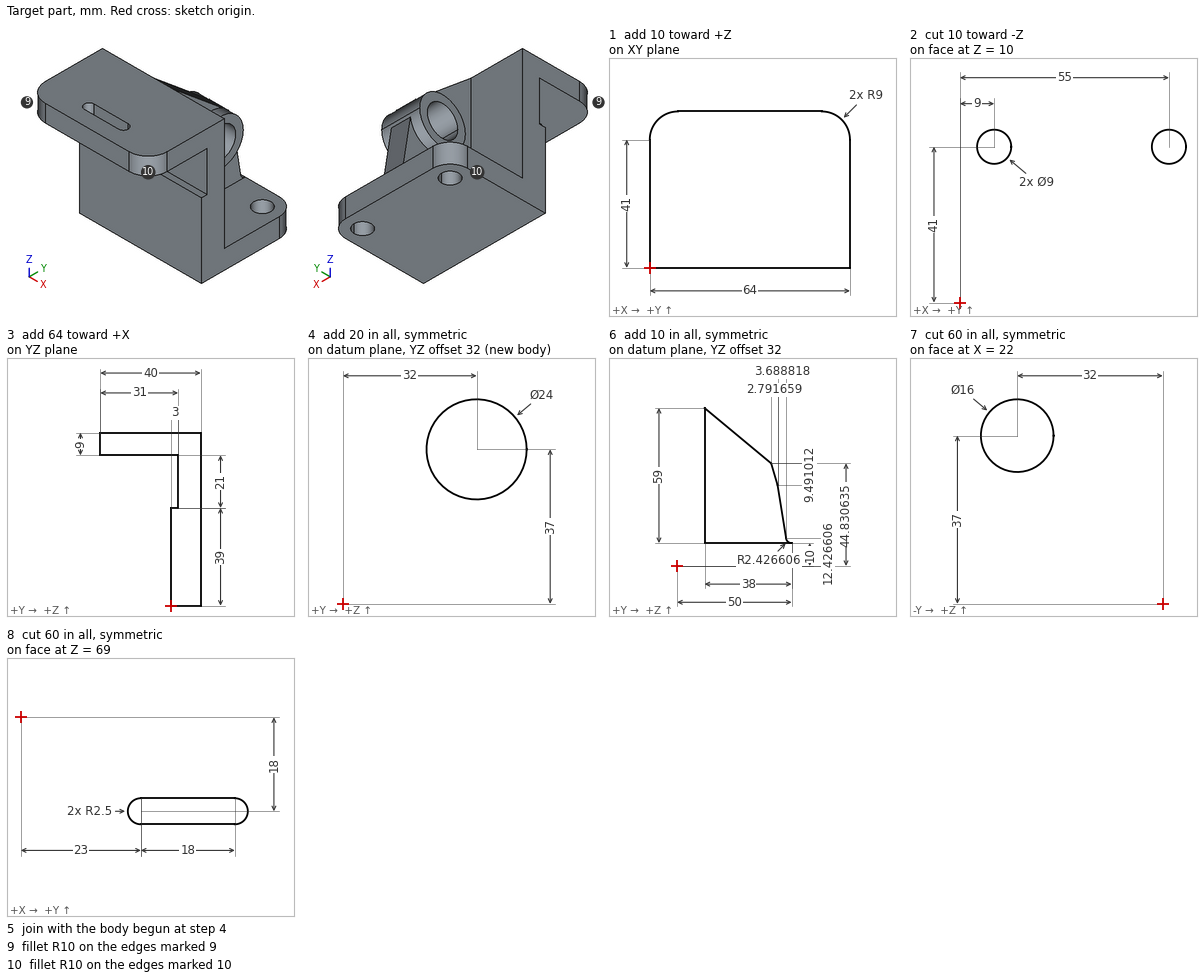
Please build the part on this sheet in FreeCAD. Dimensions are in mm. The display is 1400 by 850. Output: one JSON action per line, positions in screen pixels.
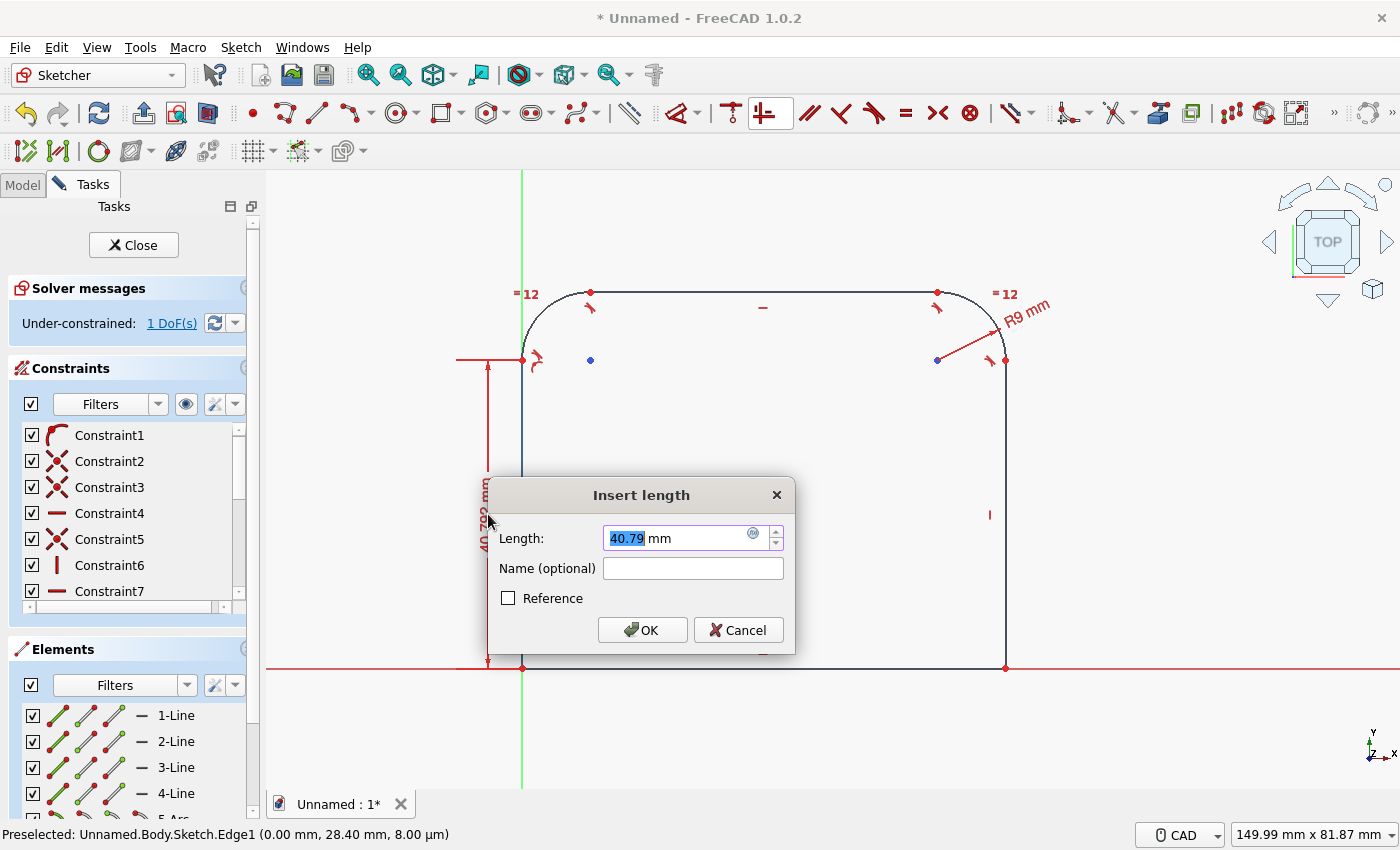
{"action": "type", "text": "41"}
{"action": "key", "text": "Return"}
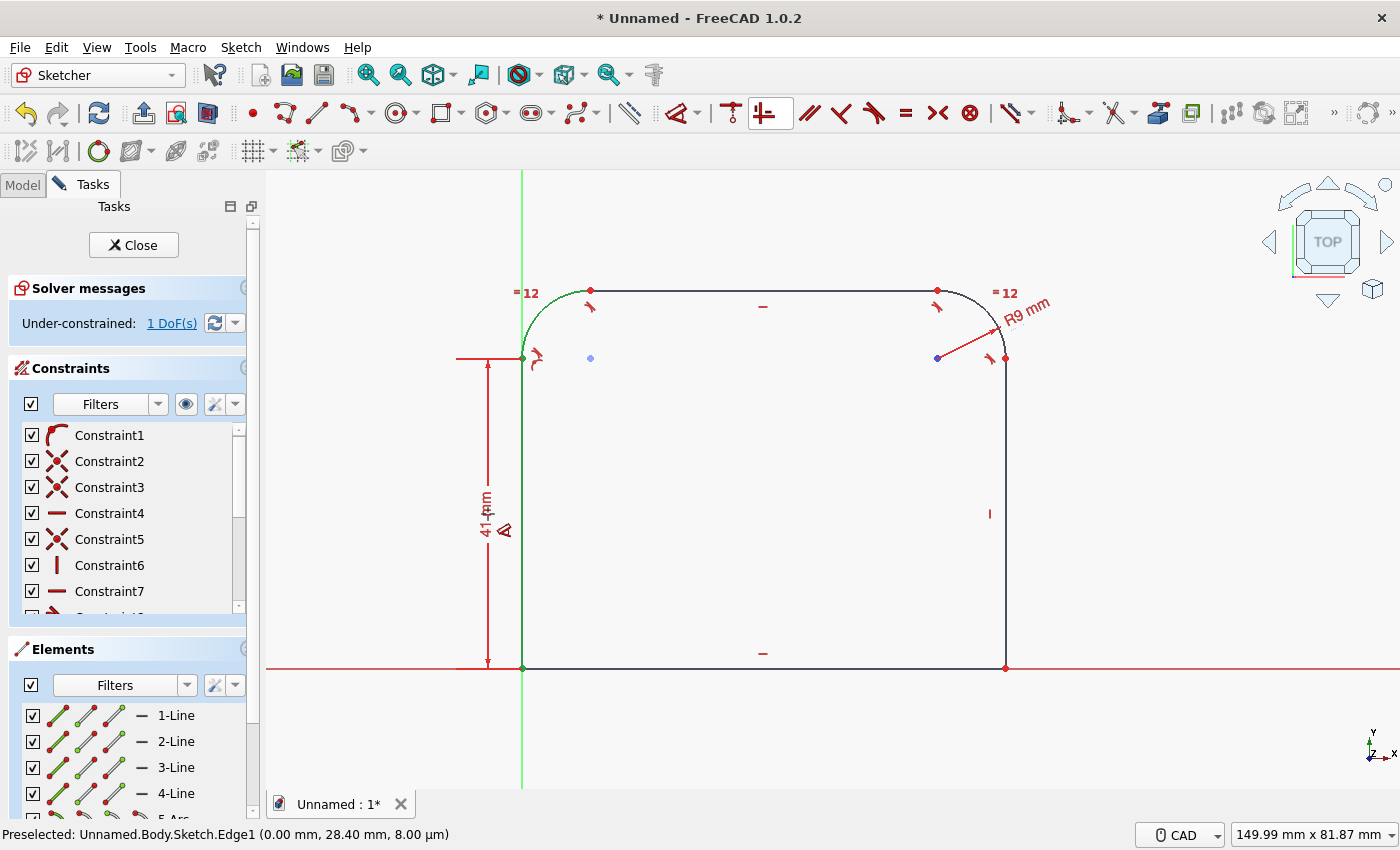
{"action": "left_click", "coordinate": [667, 669]}
{"action": "left_click", "coordinate": [764, 703]}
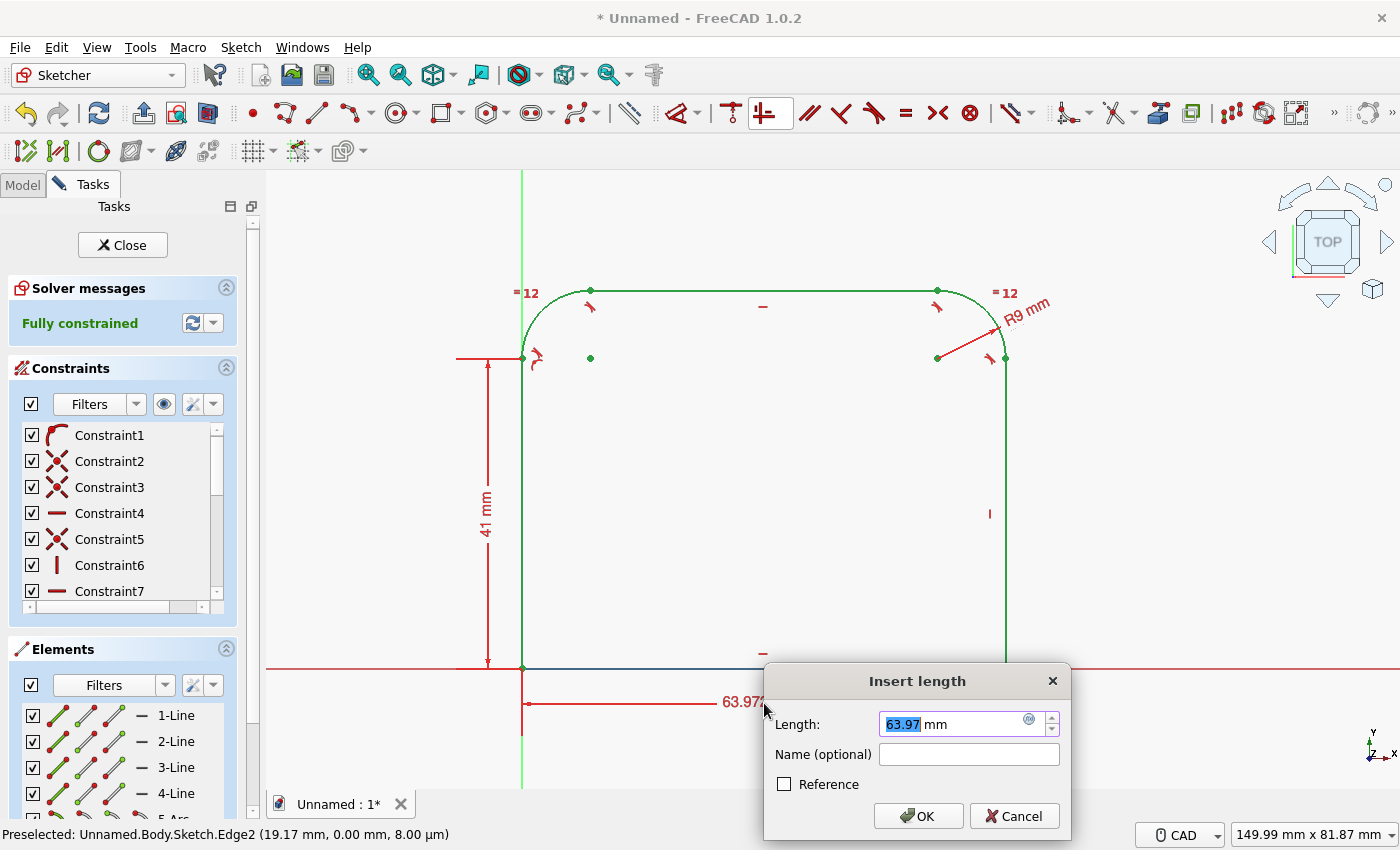
{"action": "type", "text": "64"}
{"action": "key", "text": "Return"}
{"action": "key", "text": "Escape"}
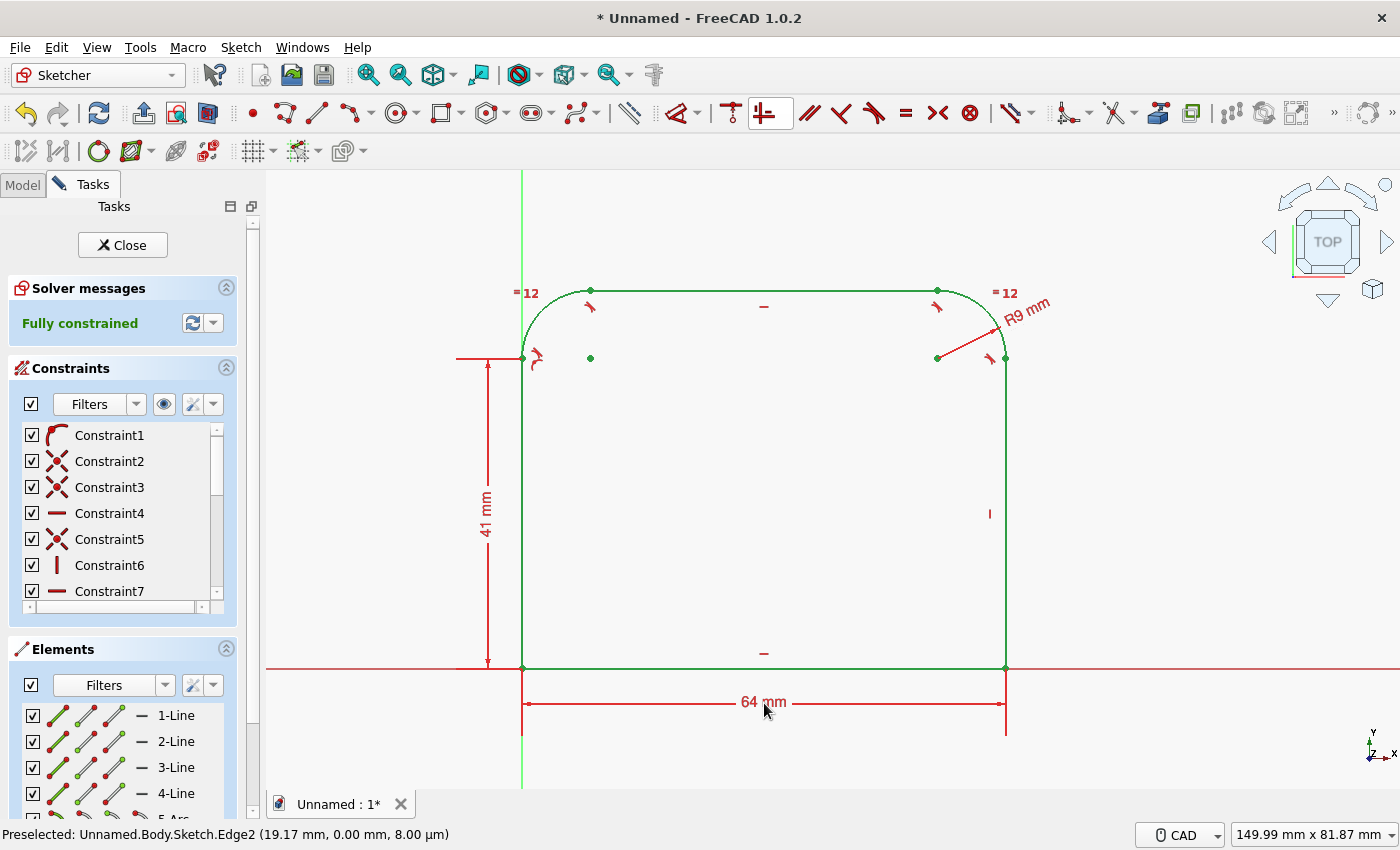
{"action": "left_click", "coordinate": [123, 245]}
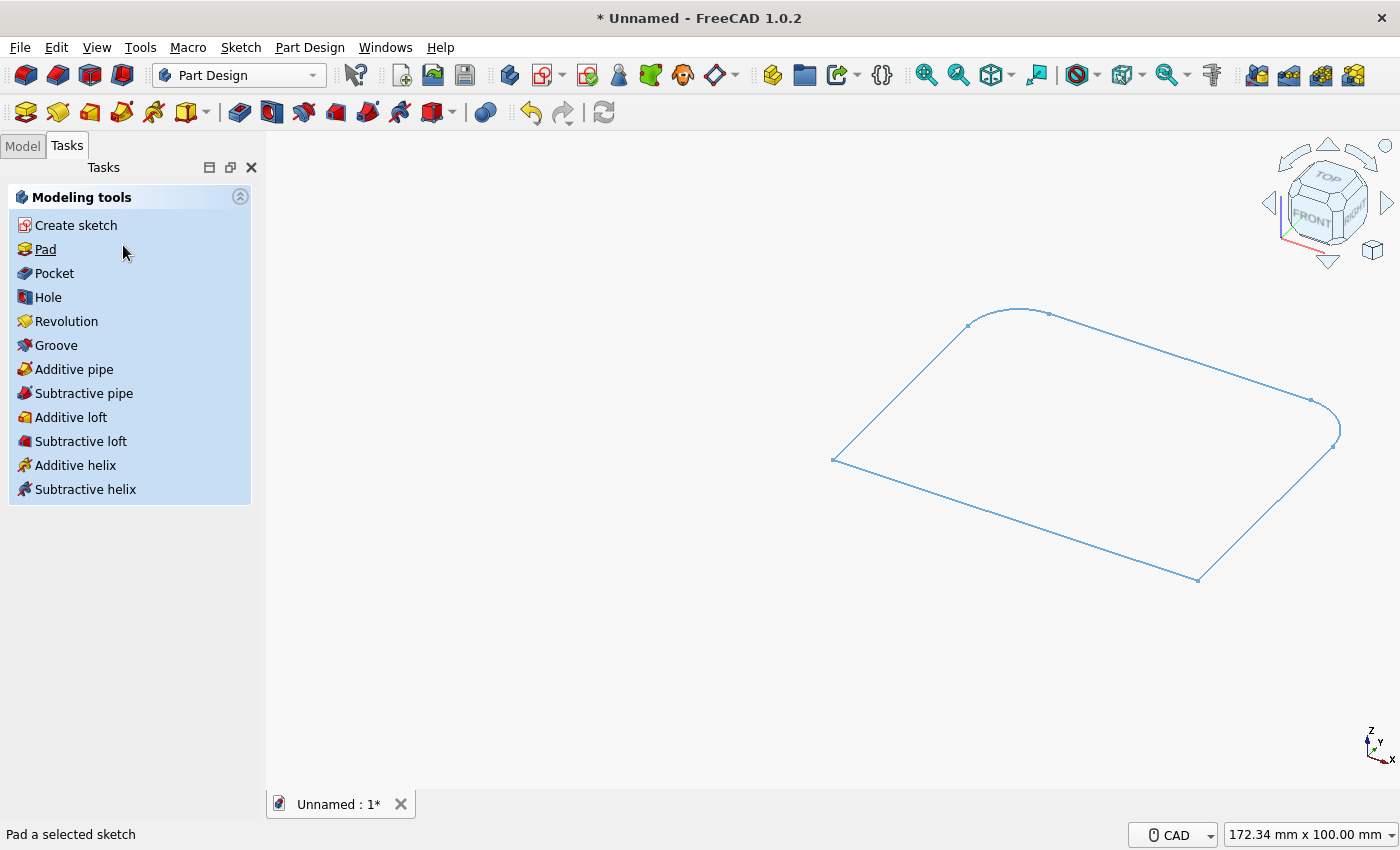
{"action": "left_click", "coordinate": [26, 112]}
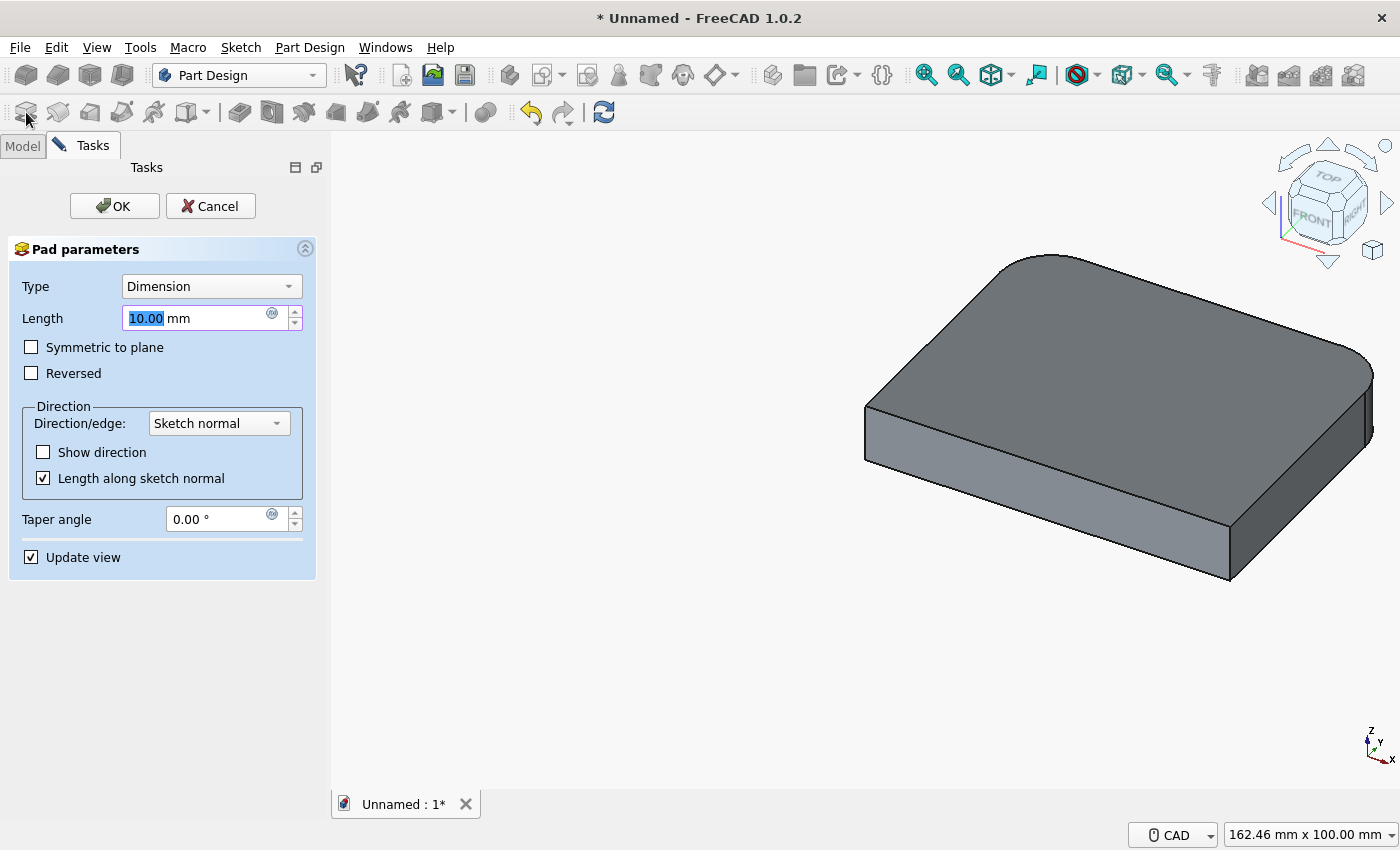
{"action": "type", "text": "10"}
{"action": "key", "text": "Tab"}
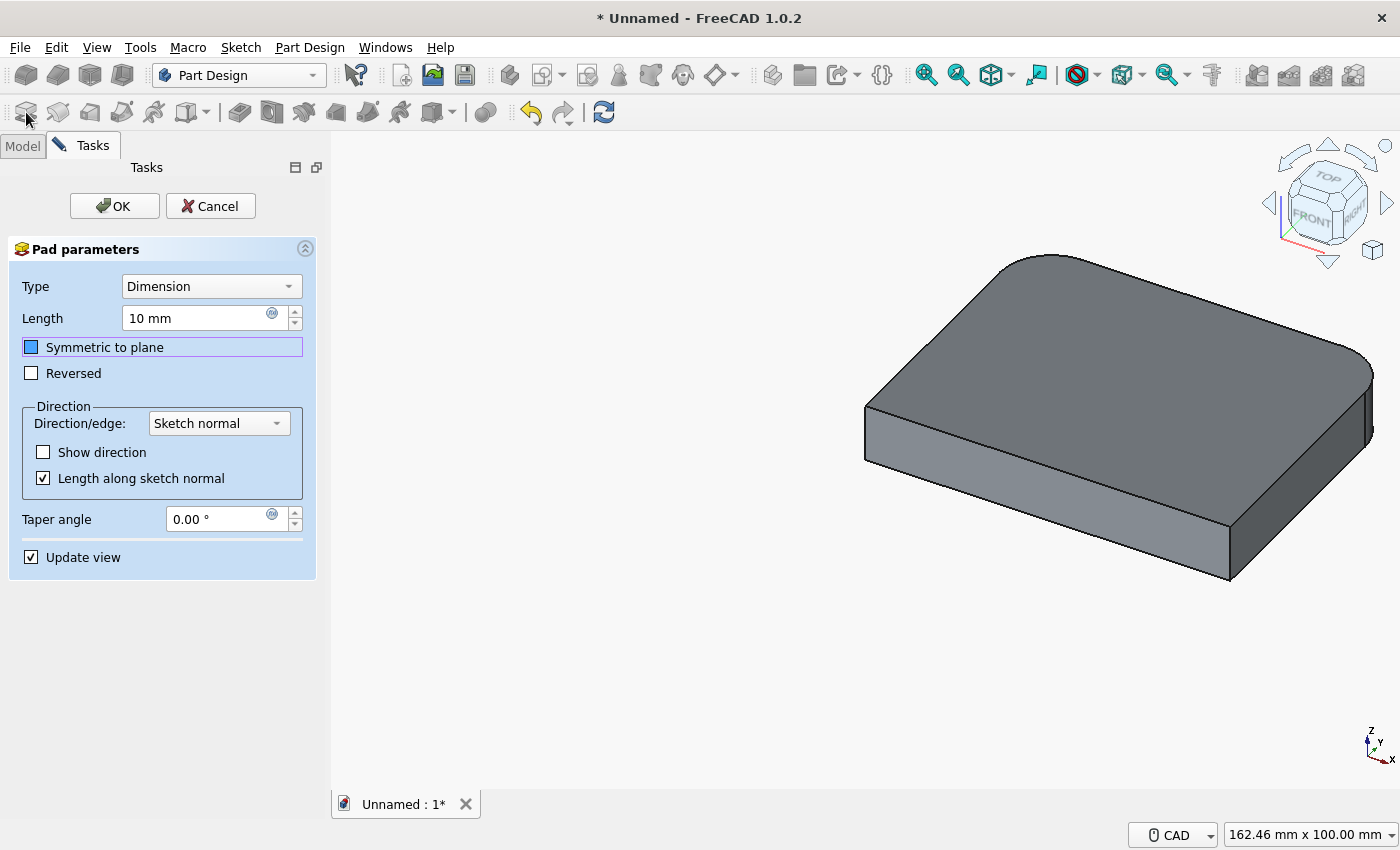
{"action": "left_click", "coordinate": [115, 206]}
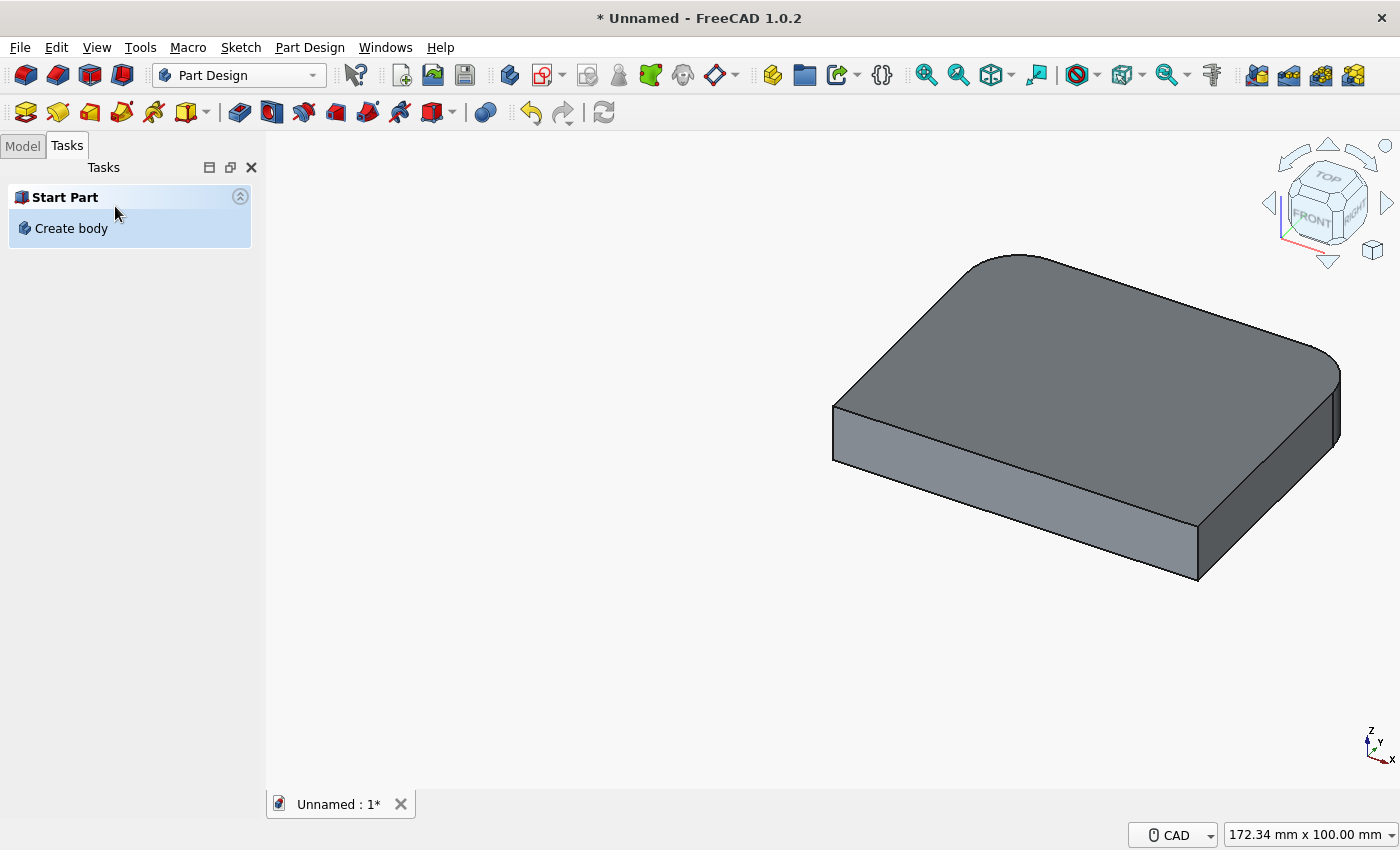
{"action": "left_click", "coordinate": [1098, 384]}